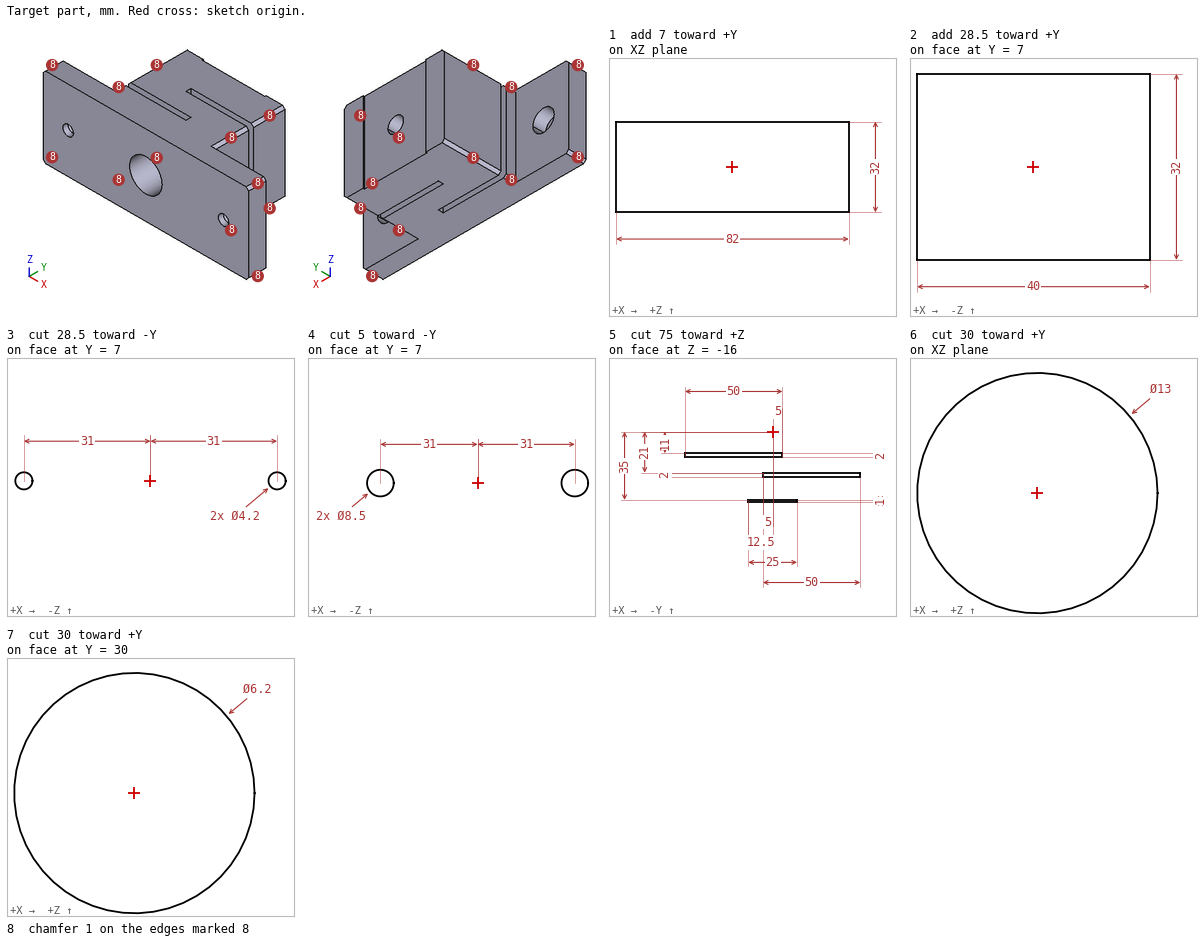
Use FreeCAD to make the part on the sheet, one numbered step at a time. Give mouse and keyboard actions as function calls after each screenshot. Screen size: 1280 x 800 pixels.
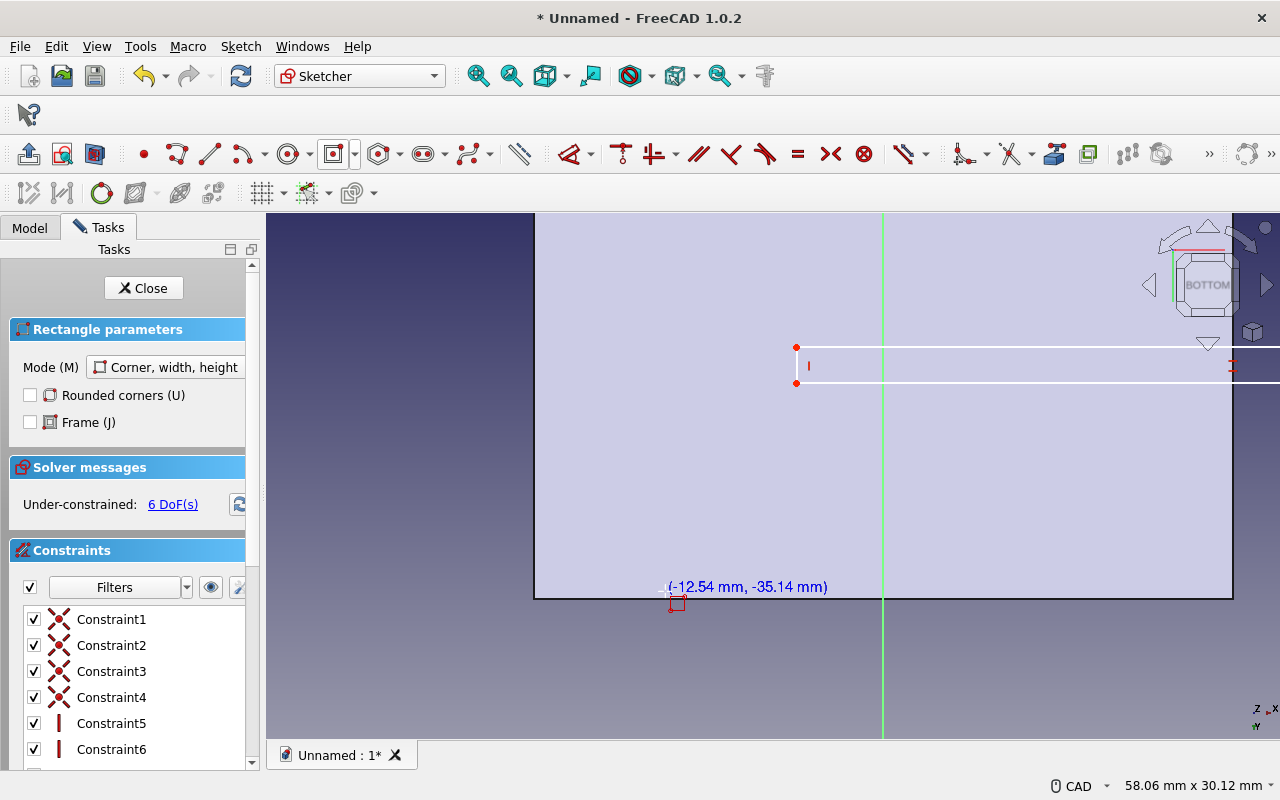
click(665, 590)
move(1102, 608)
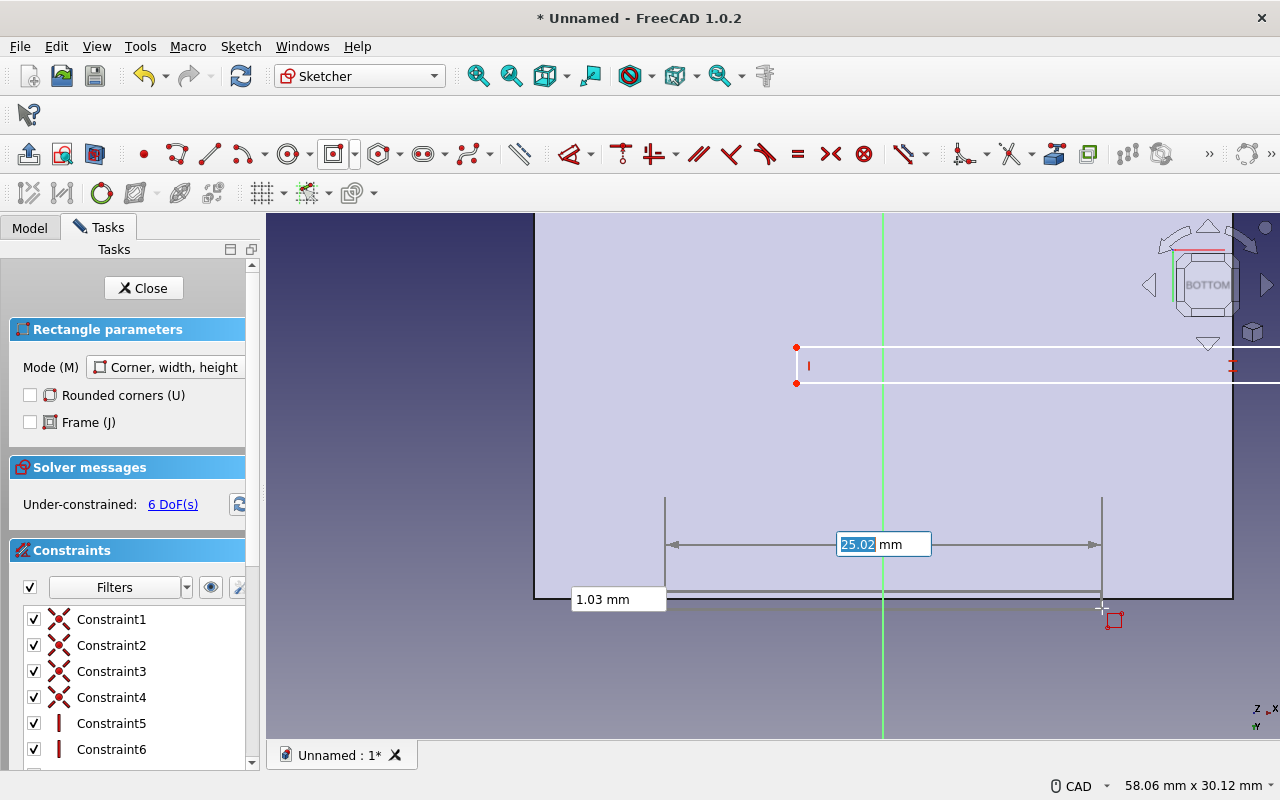
text(25)
key(Tab)
text(1)
key(Return)
key(Escape)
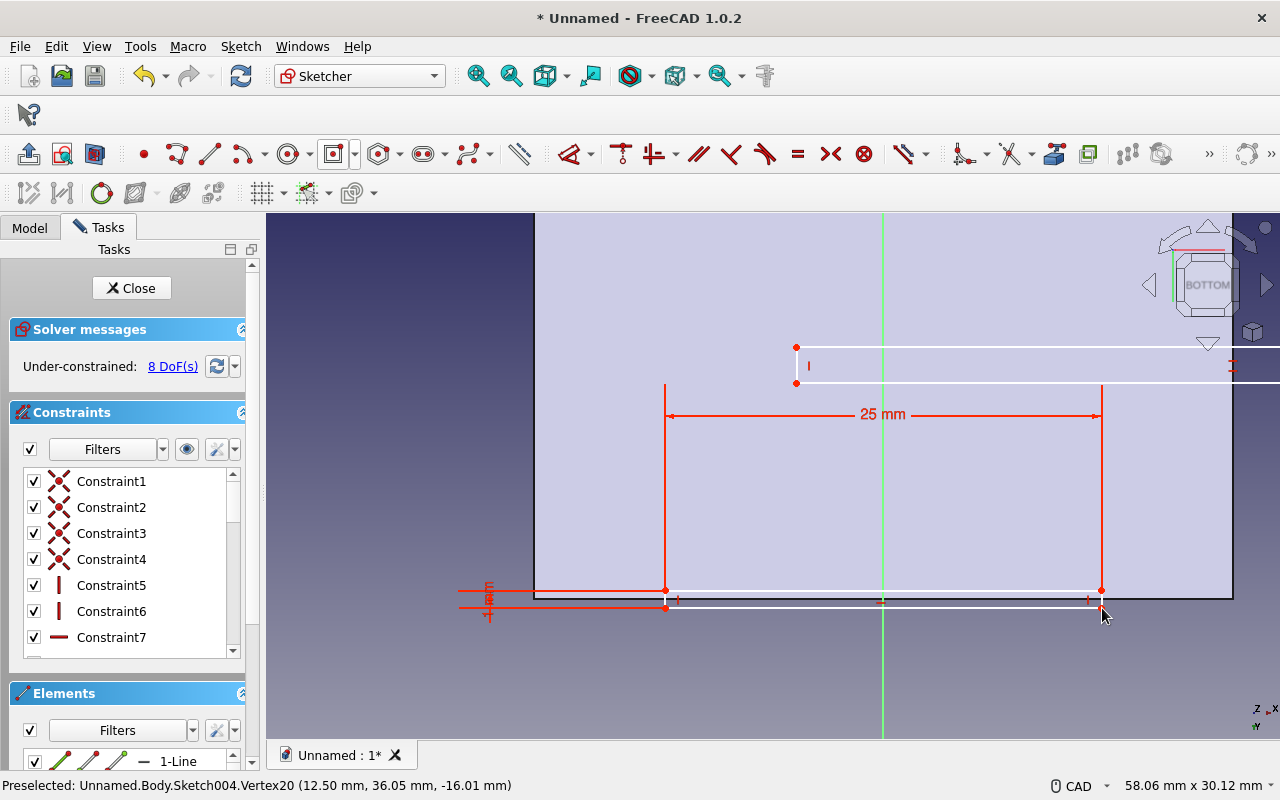
key(d)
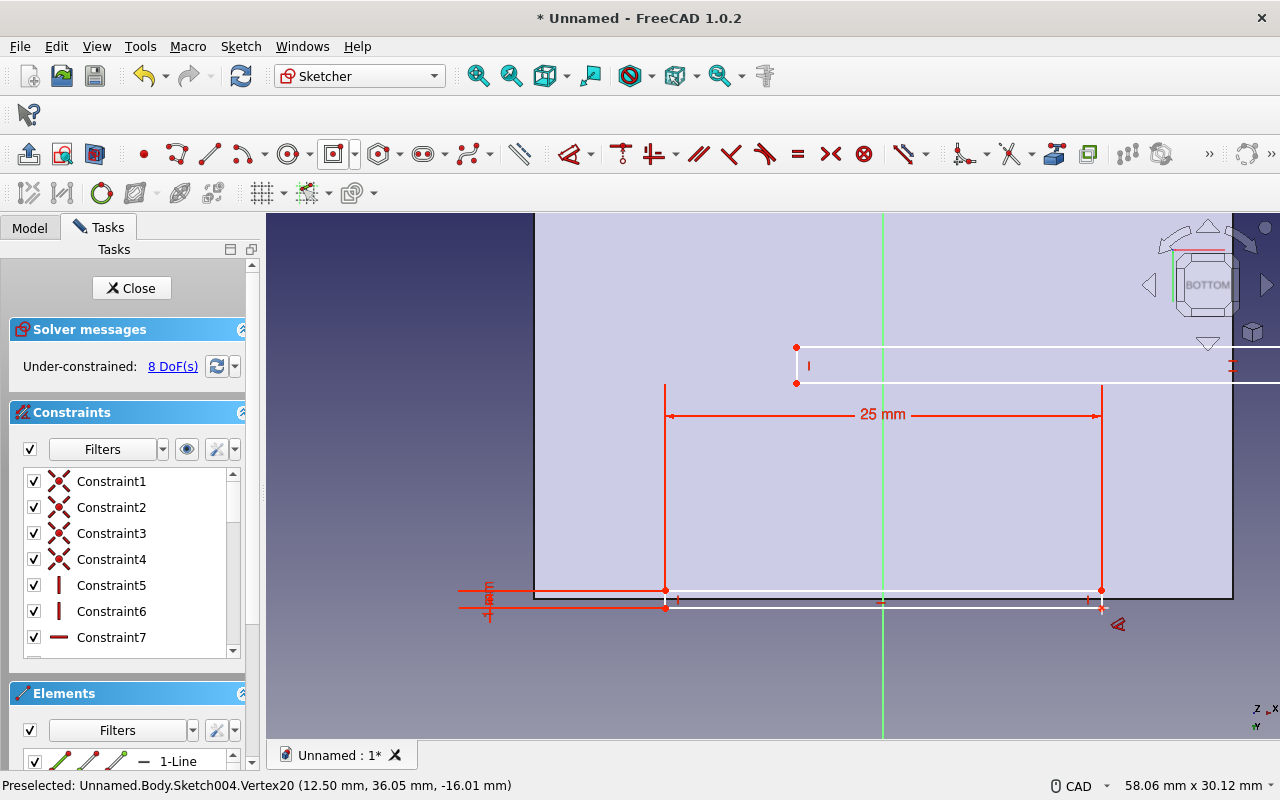
scroll(797, 358, up, 2)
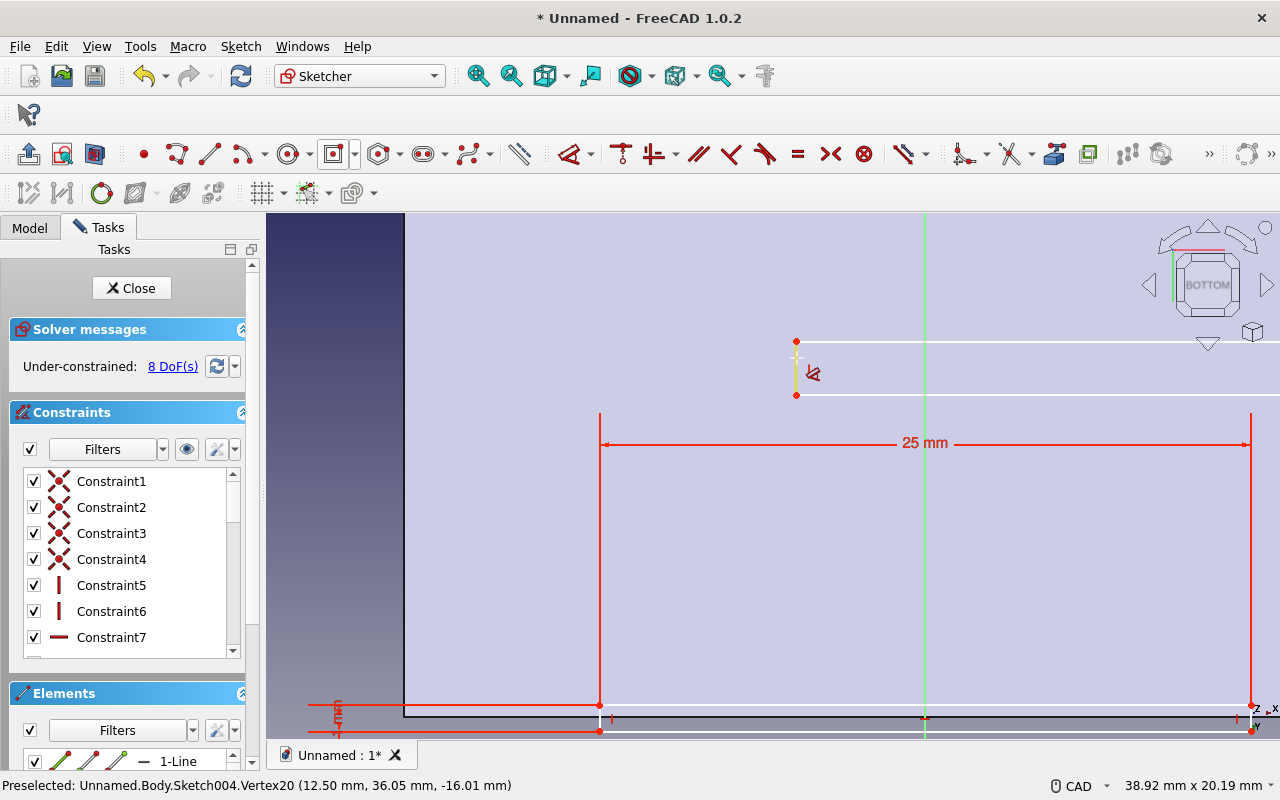
click(796, 358)
click(762, 369)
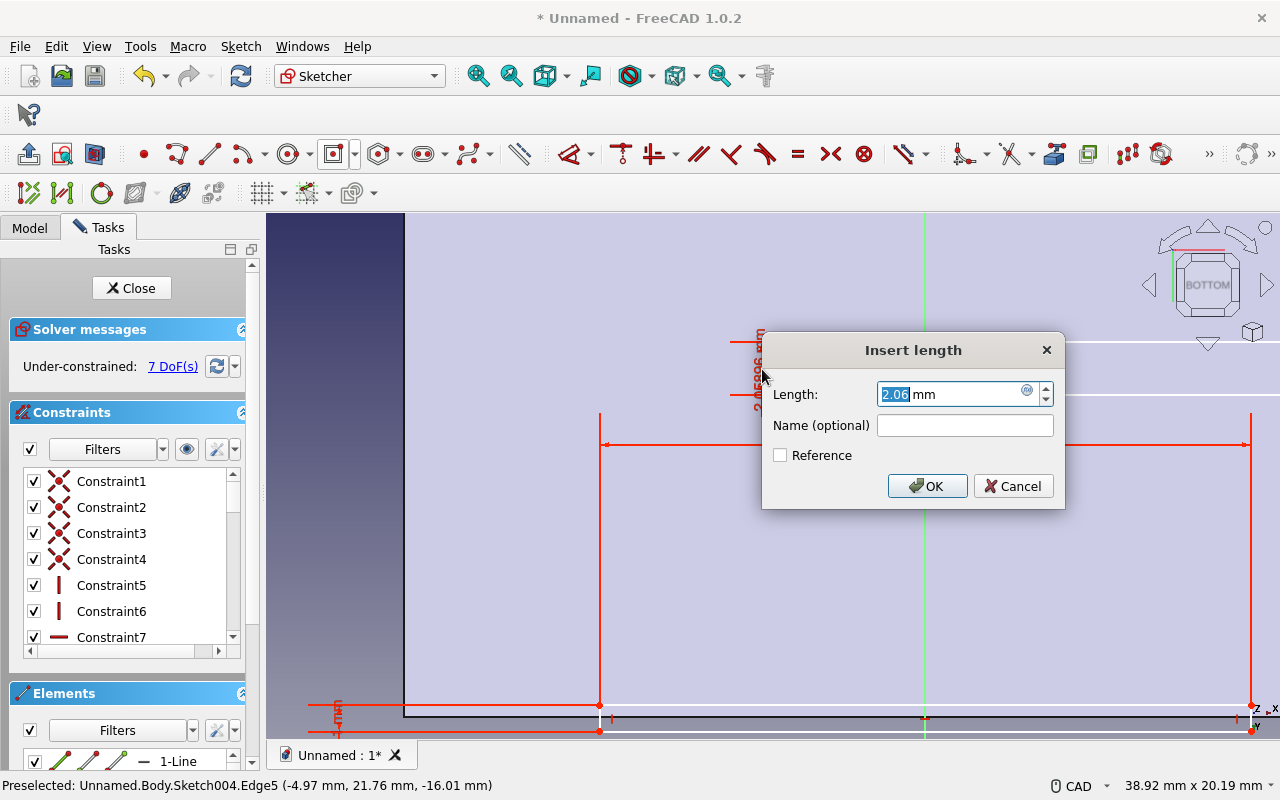
text(2)
key(Return)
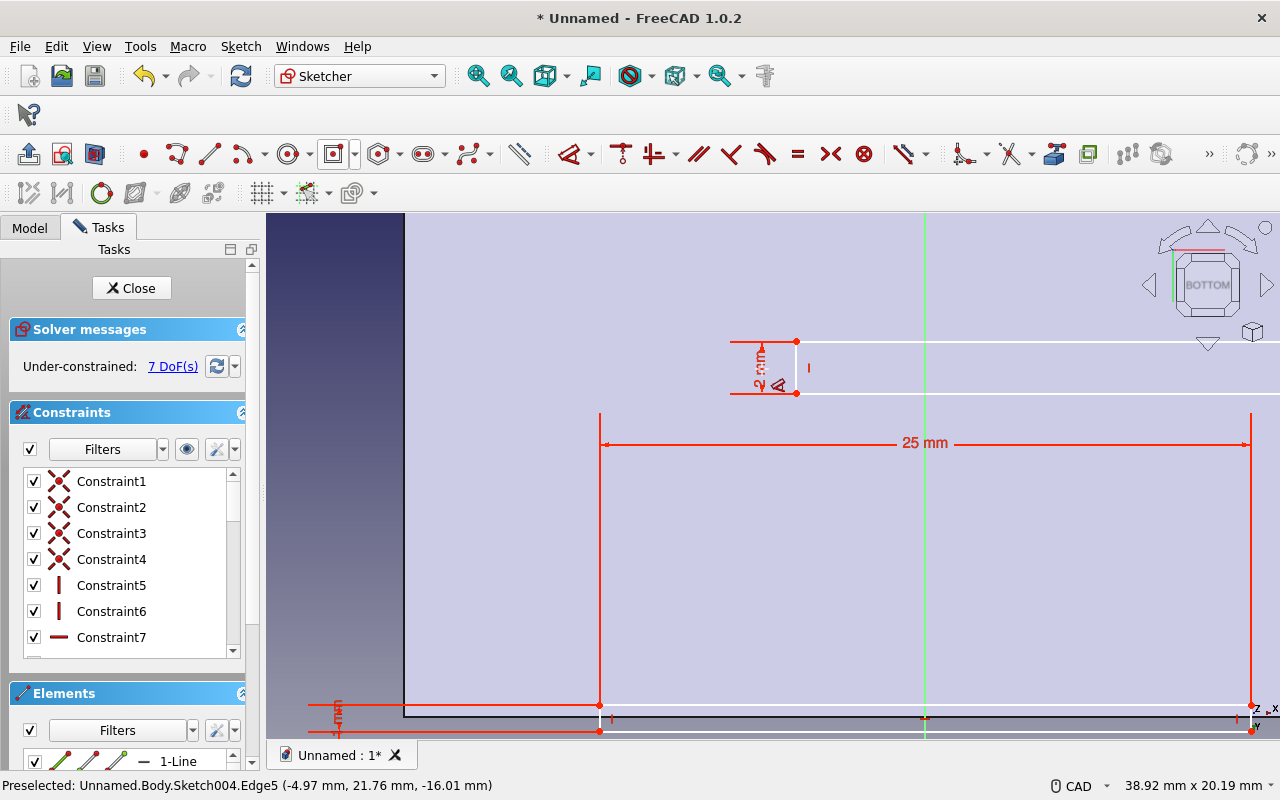
scroll(632, 546, down, 7)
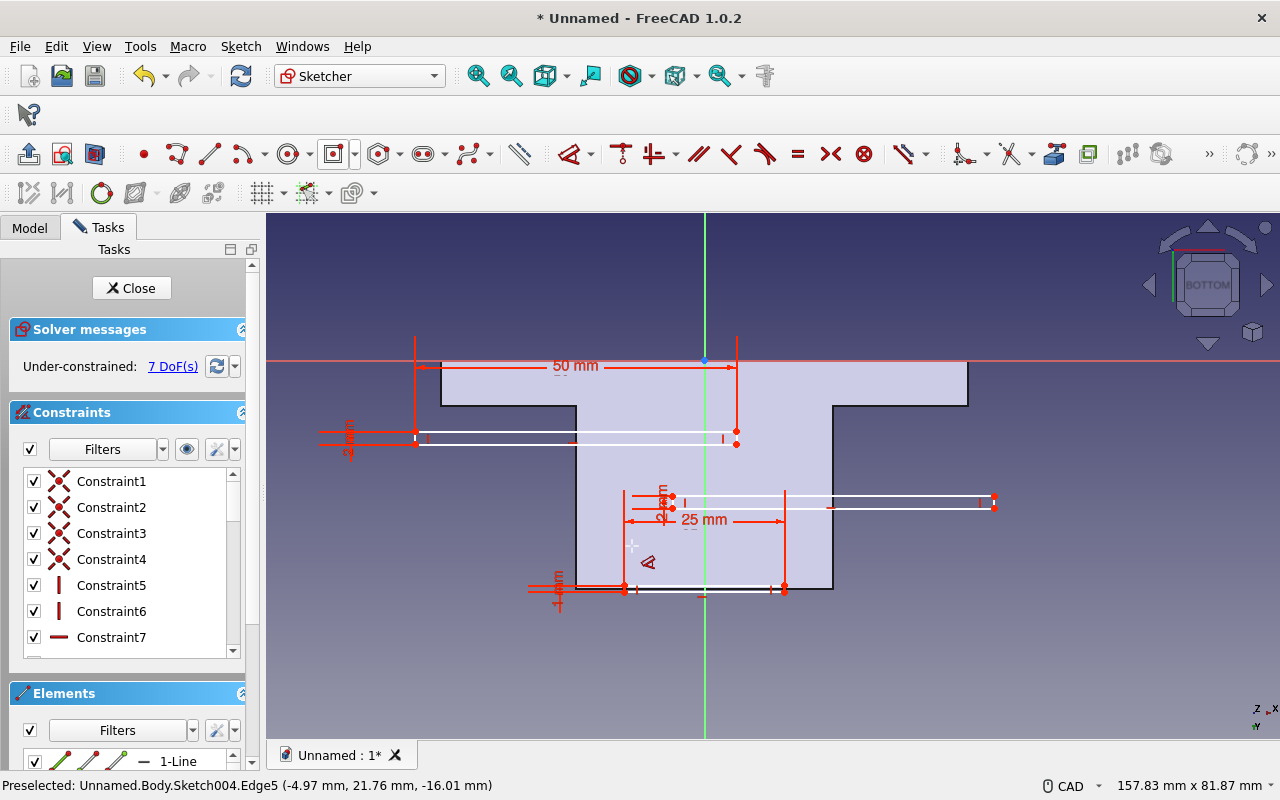
click(737, 509)
click(833, 543)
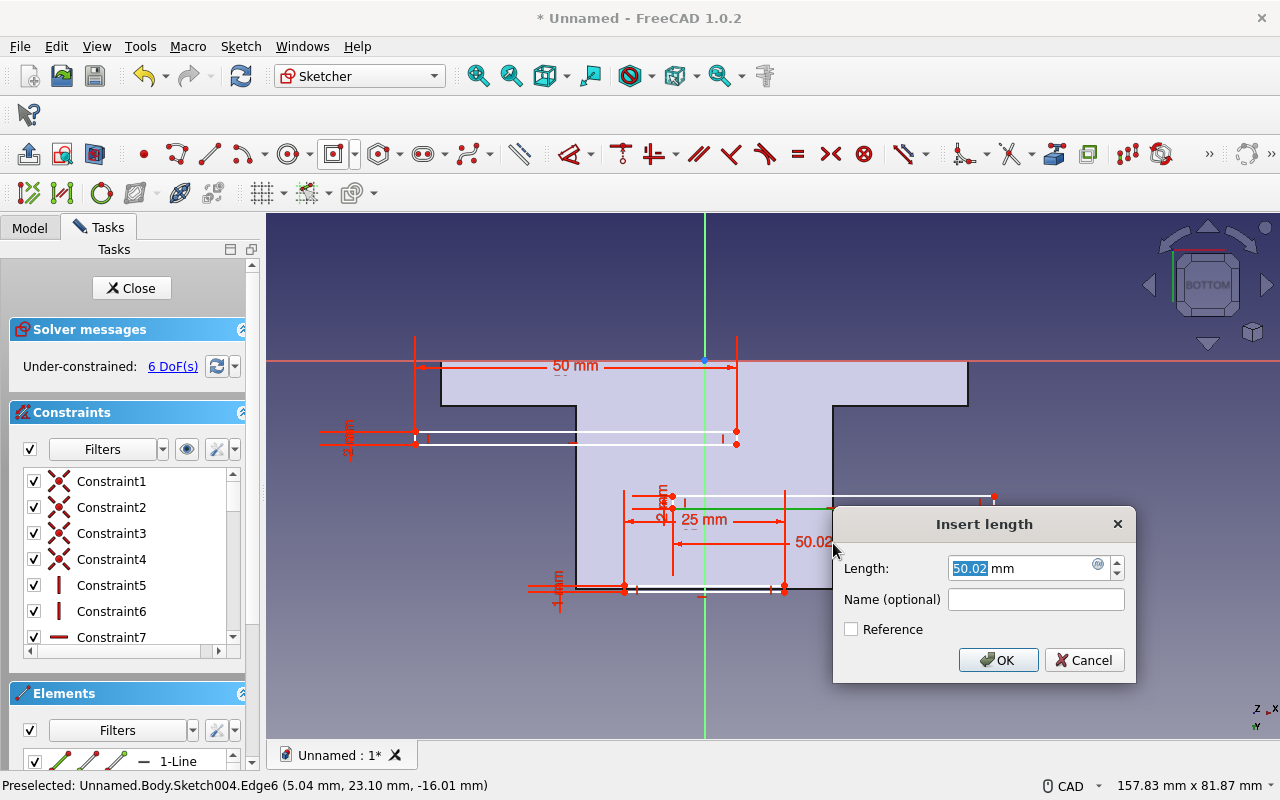
text(50)
key(Return)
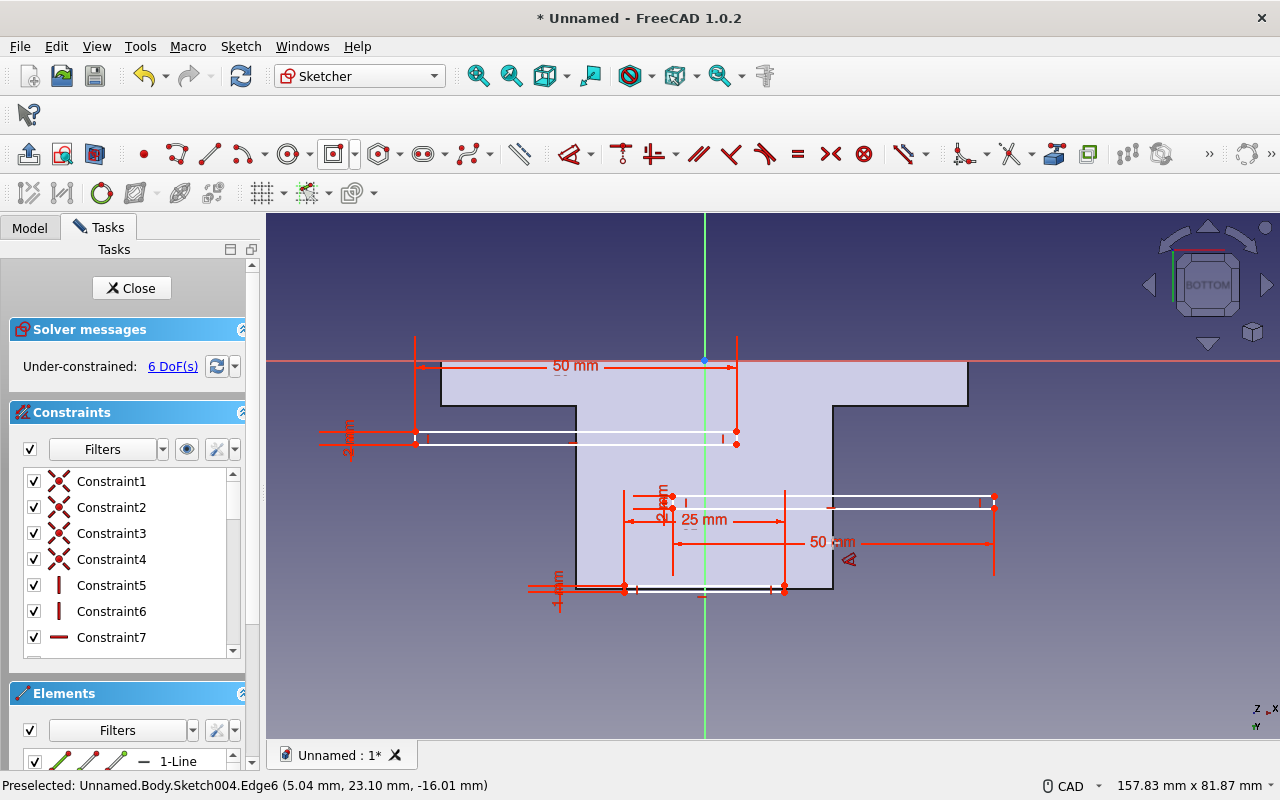
scroll(737, 445, up, 2)